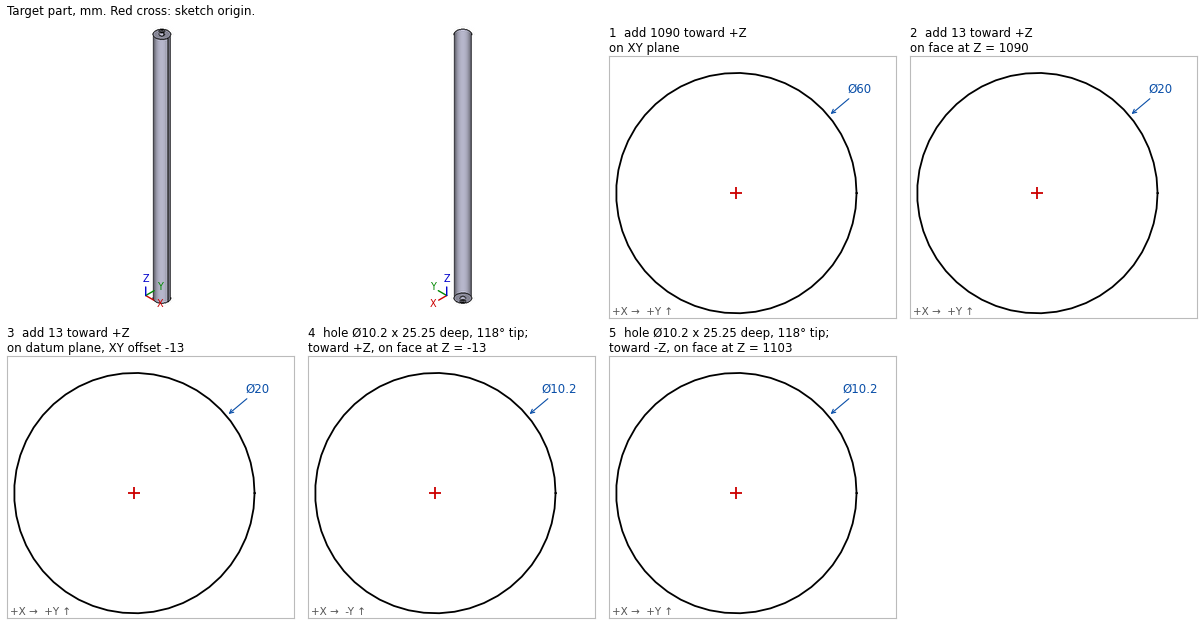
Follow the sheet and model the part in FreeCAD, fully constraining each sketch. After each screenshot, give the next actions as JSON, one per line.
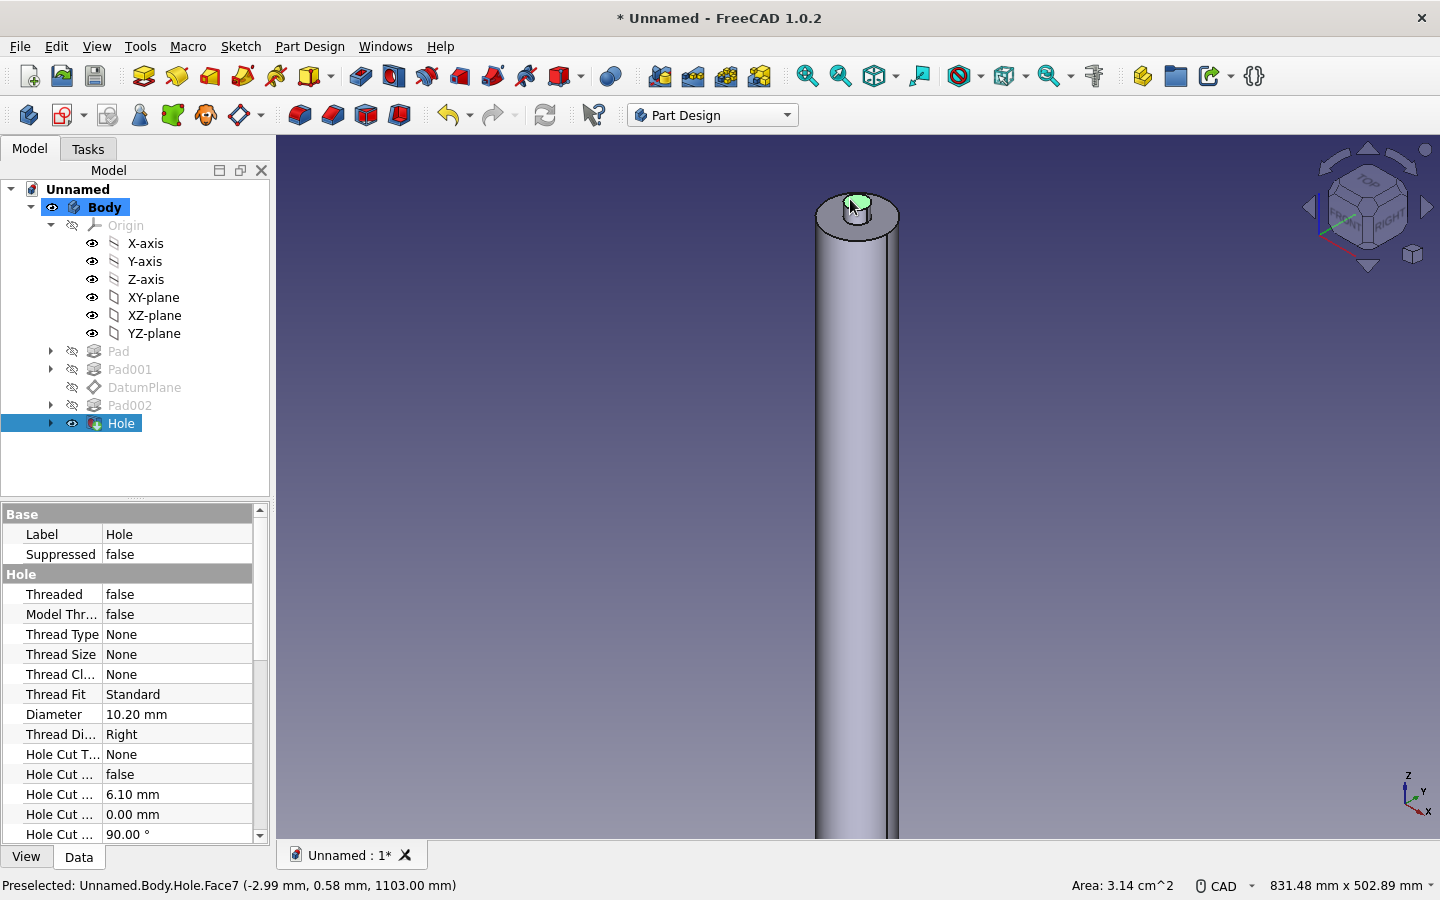
{"action": "left_click", "coordinate": [62, 116]}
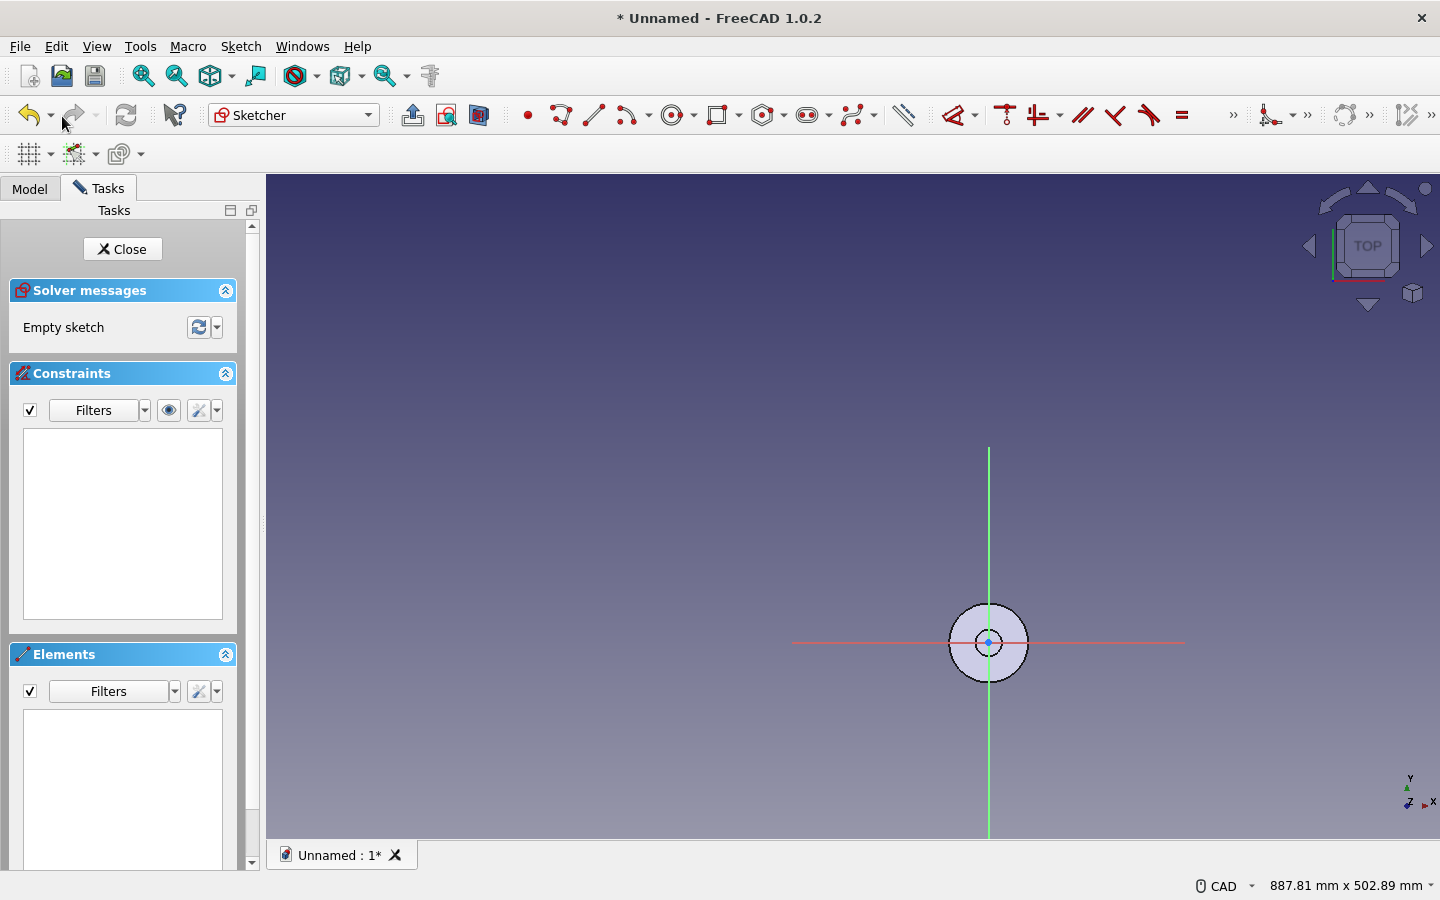
{"action": "scroll", "coordinate": [999, 650], "scroll_direction": "up", "scroll_amount": 15}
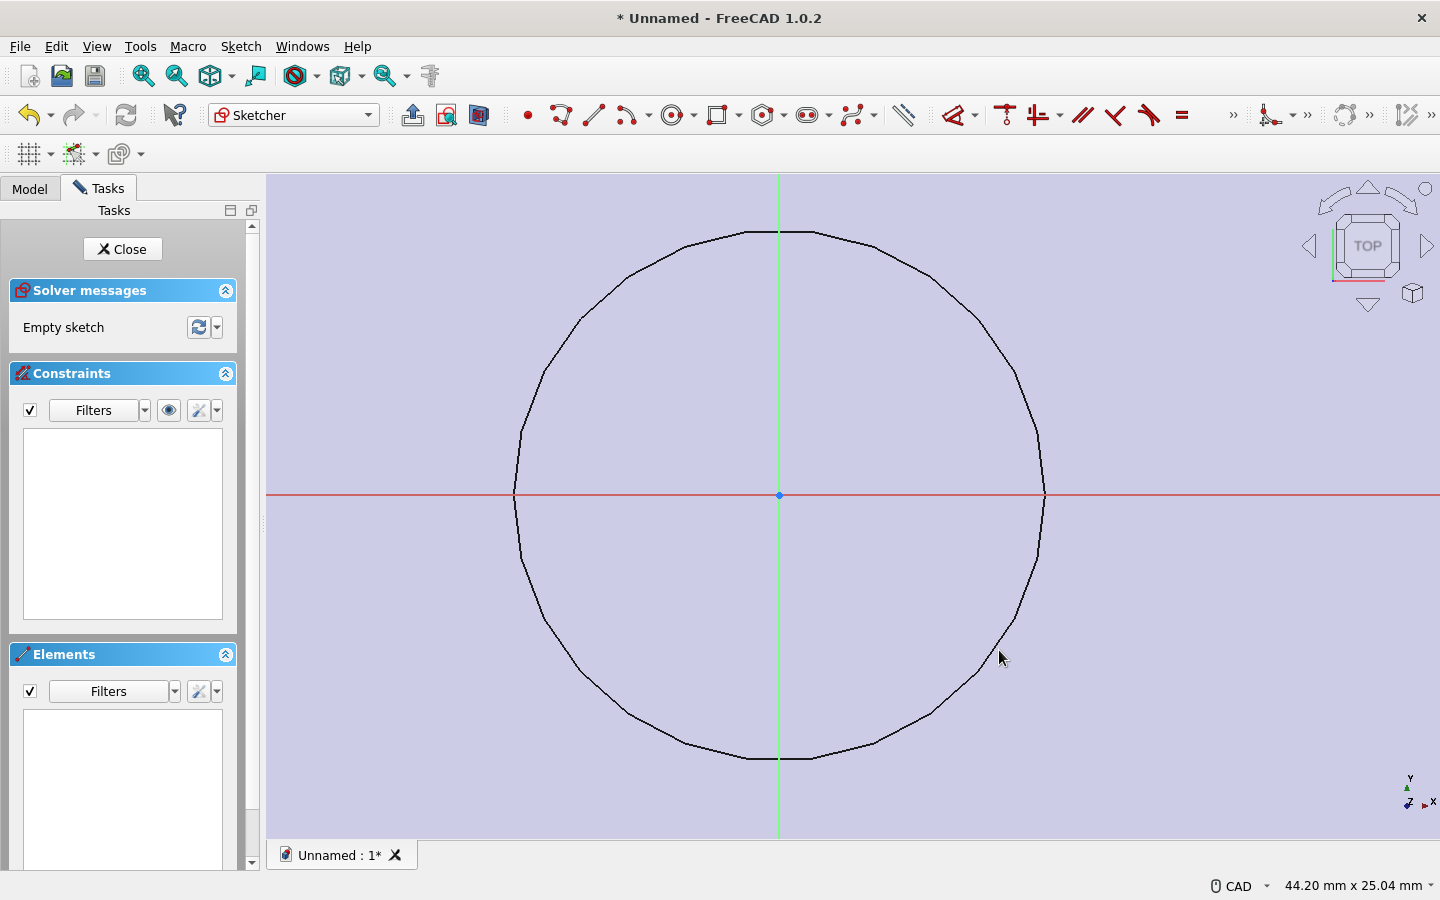
{"action": "scroll", "coordinate": [769, 472], "scroll_direction": "up", "scroll_amount": 2}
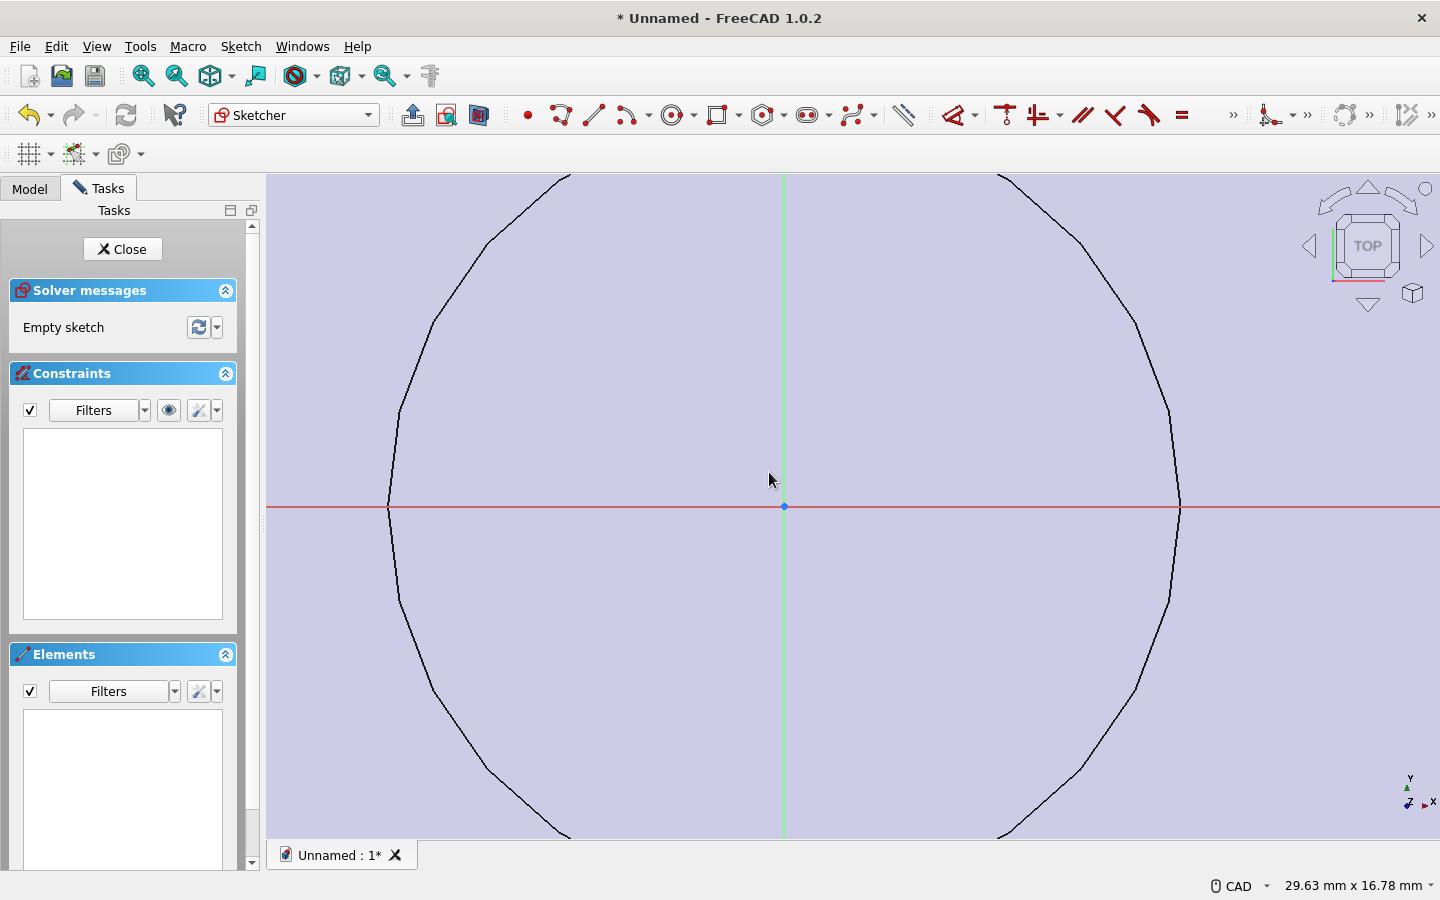
{"action": "key", "text": "g c"}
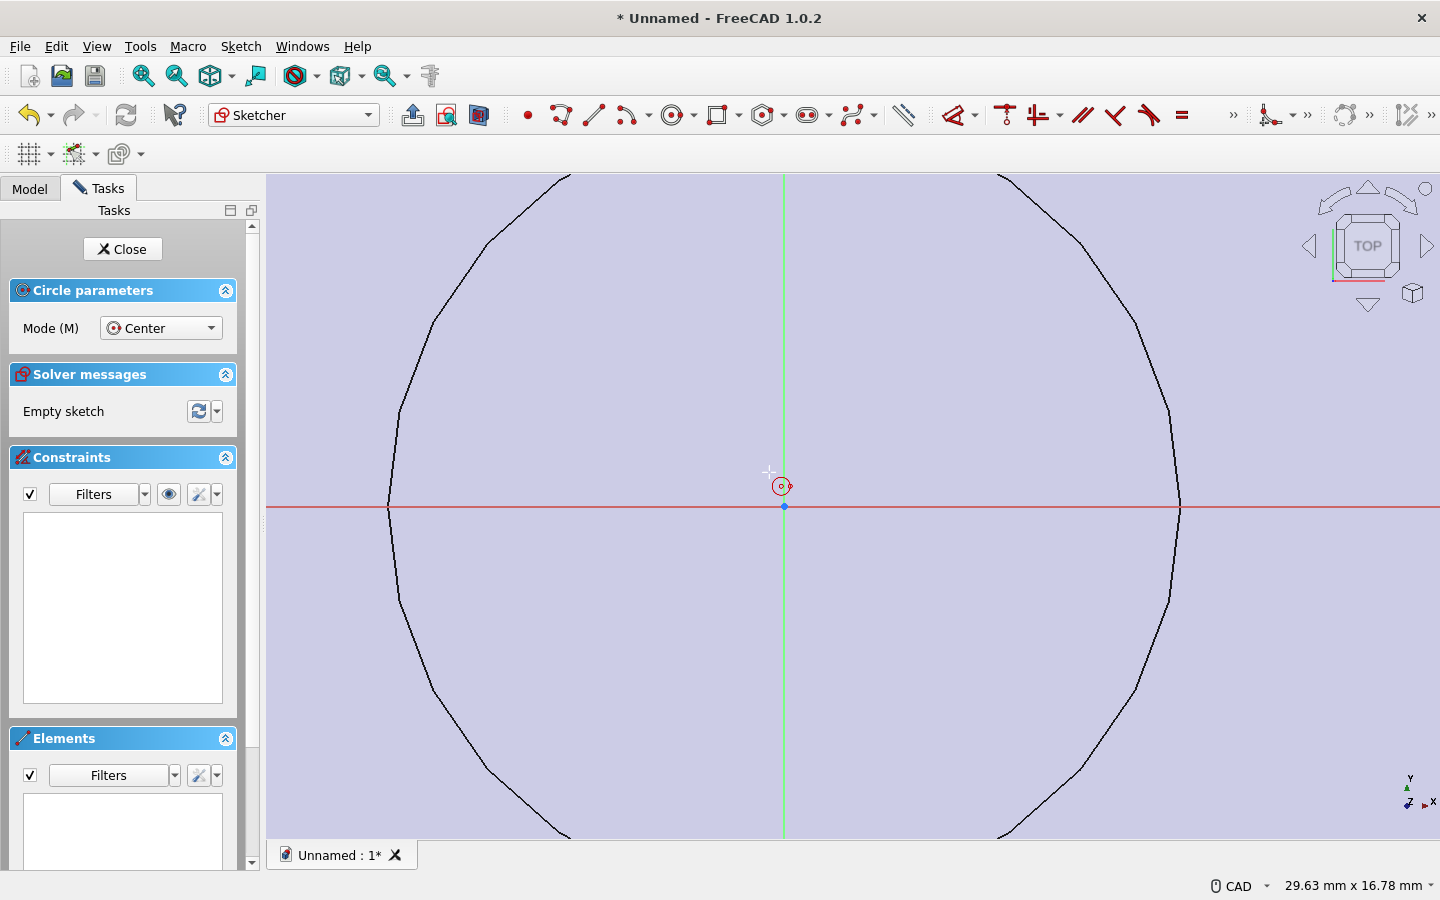
{"action": "left_click", "coordinate": [784, 507]}
{"action": "mouse_move", "coordinate": [927, 364]}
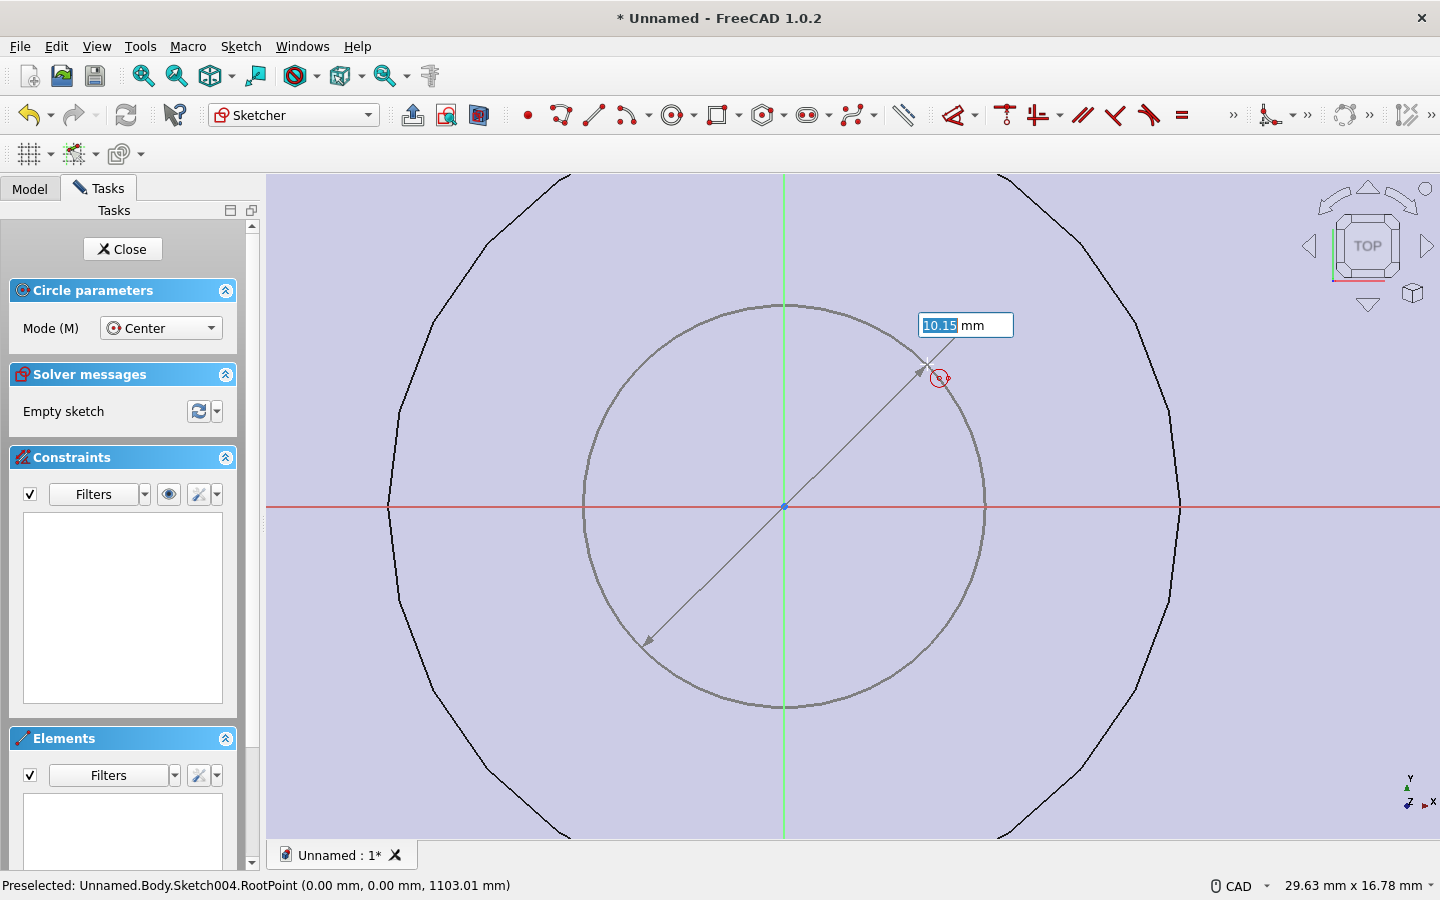
{"action": "type", "text": "10.2"}
{"action": "key", "text": "Return"}
{"action": "key", "text": "Escape"}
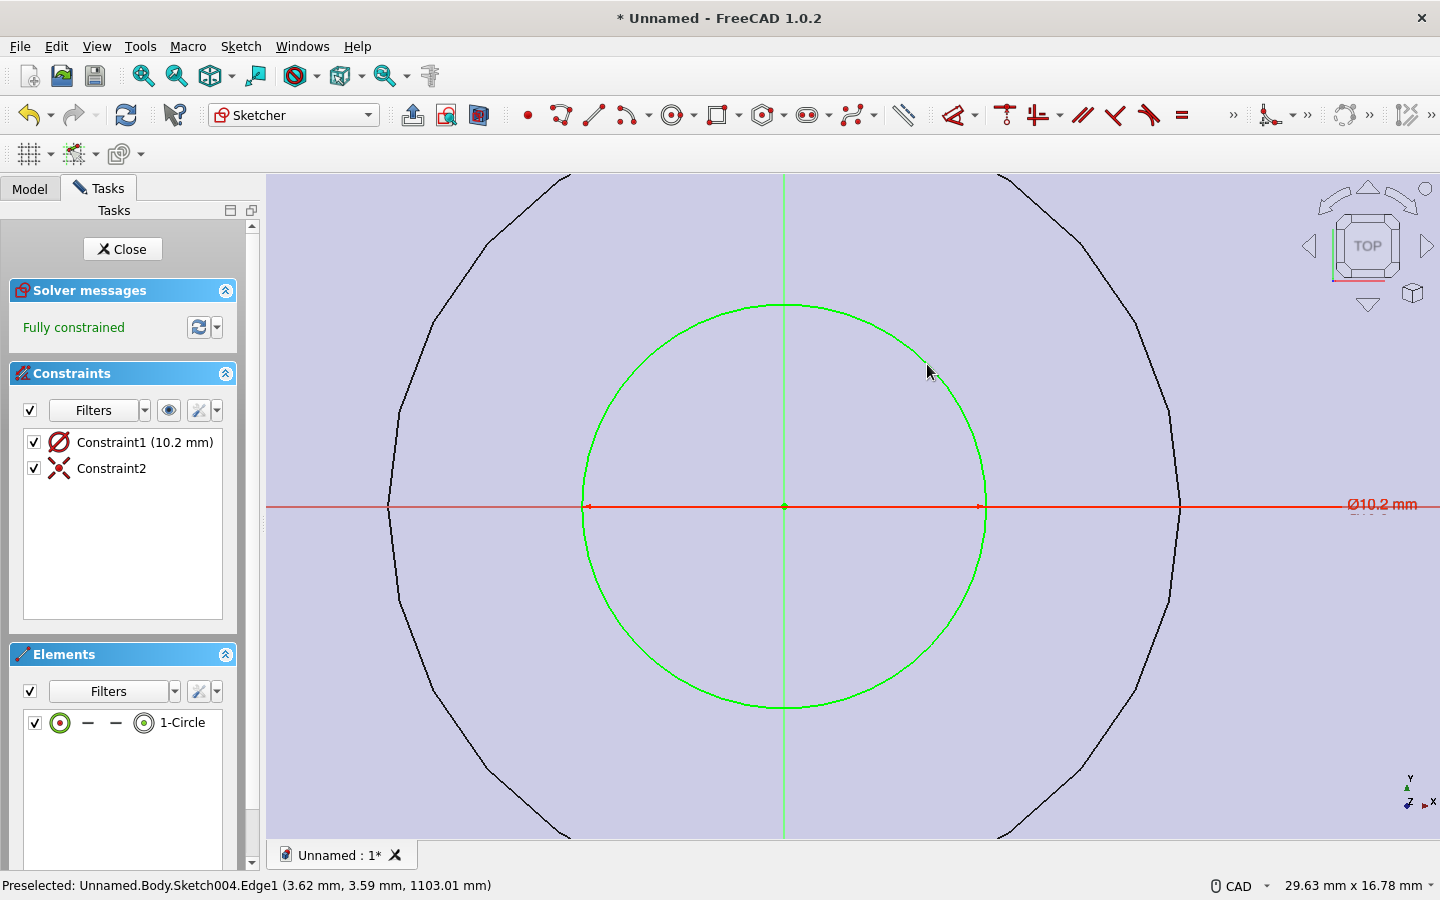
{"action": "left_click", "coordinate": [123, 249]}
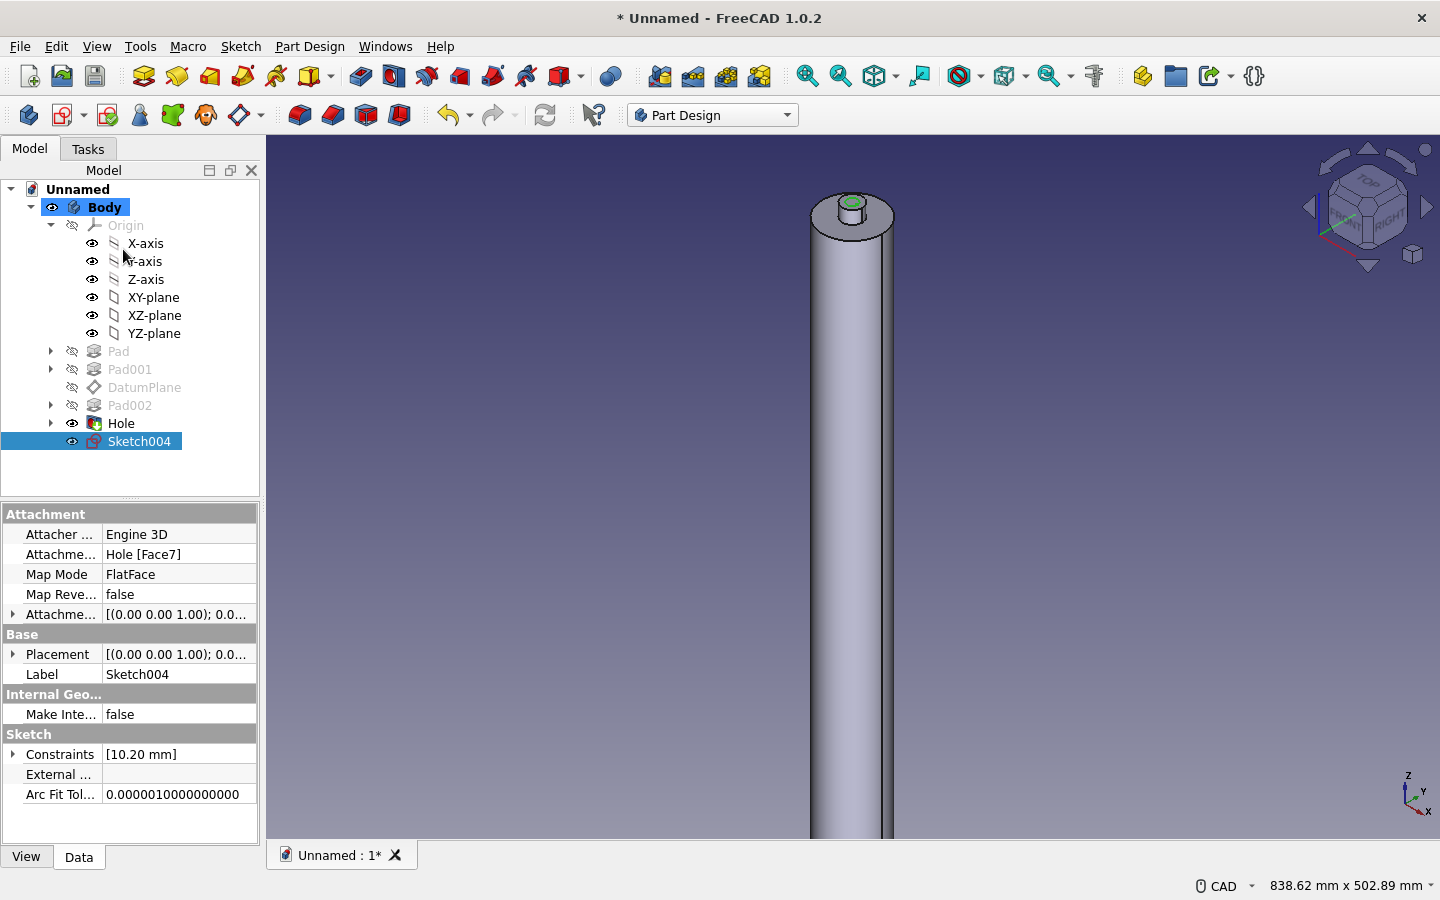
{"action": "left_click", "coordinate": [394, 76]}